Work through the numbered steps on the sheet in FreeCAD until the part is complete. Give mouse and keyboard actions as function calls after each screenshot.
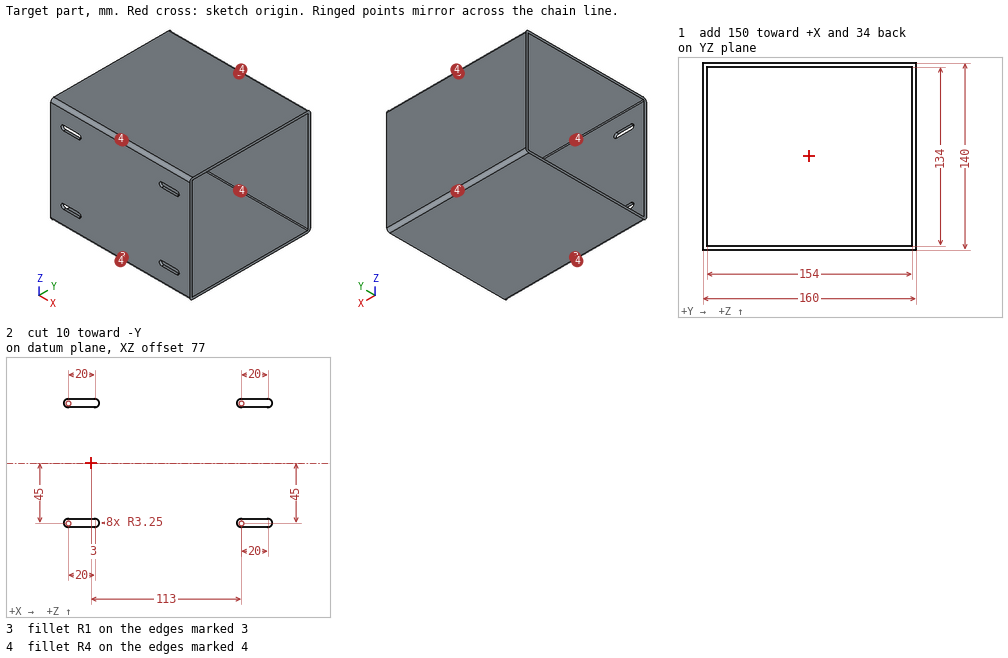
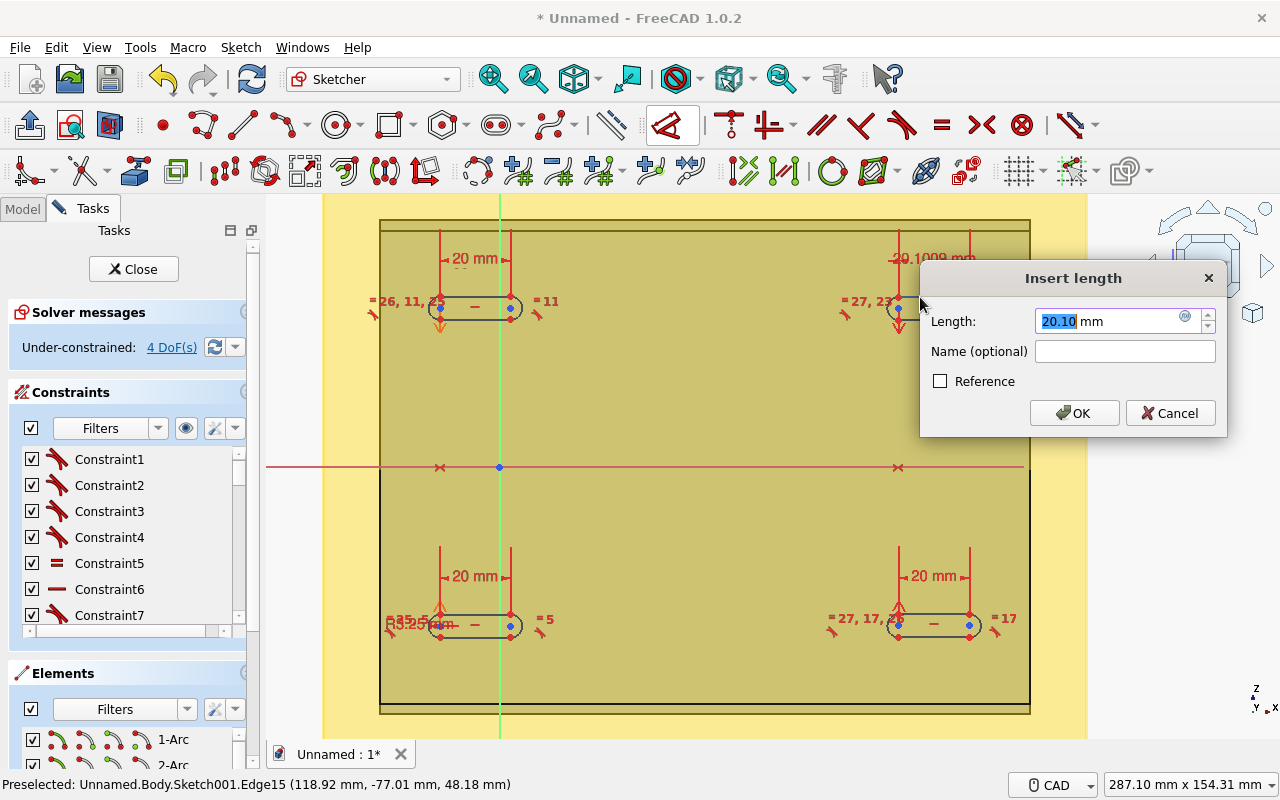
text(20)
key(Return)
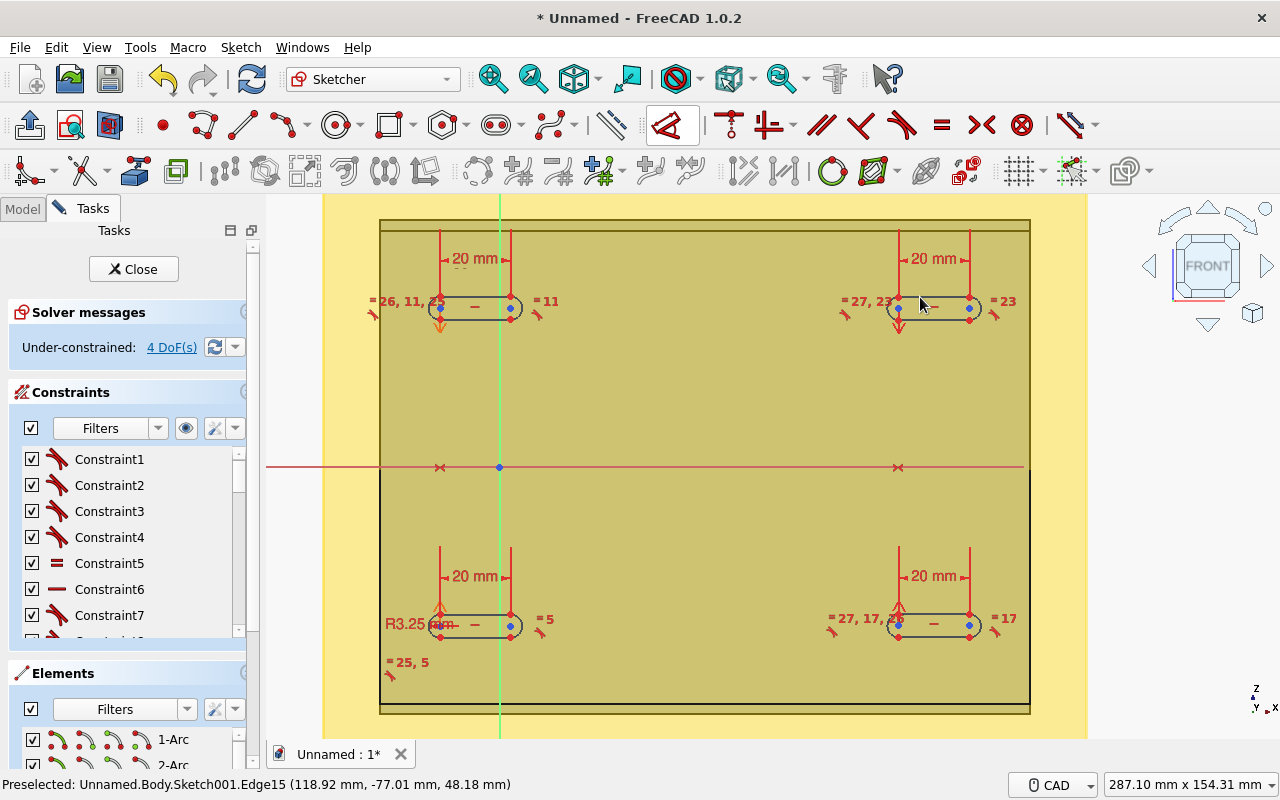
scroll(511, 638, up, 7)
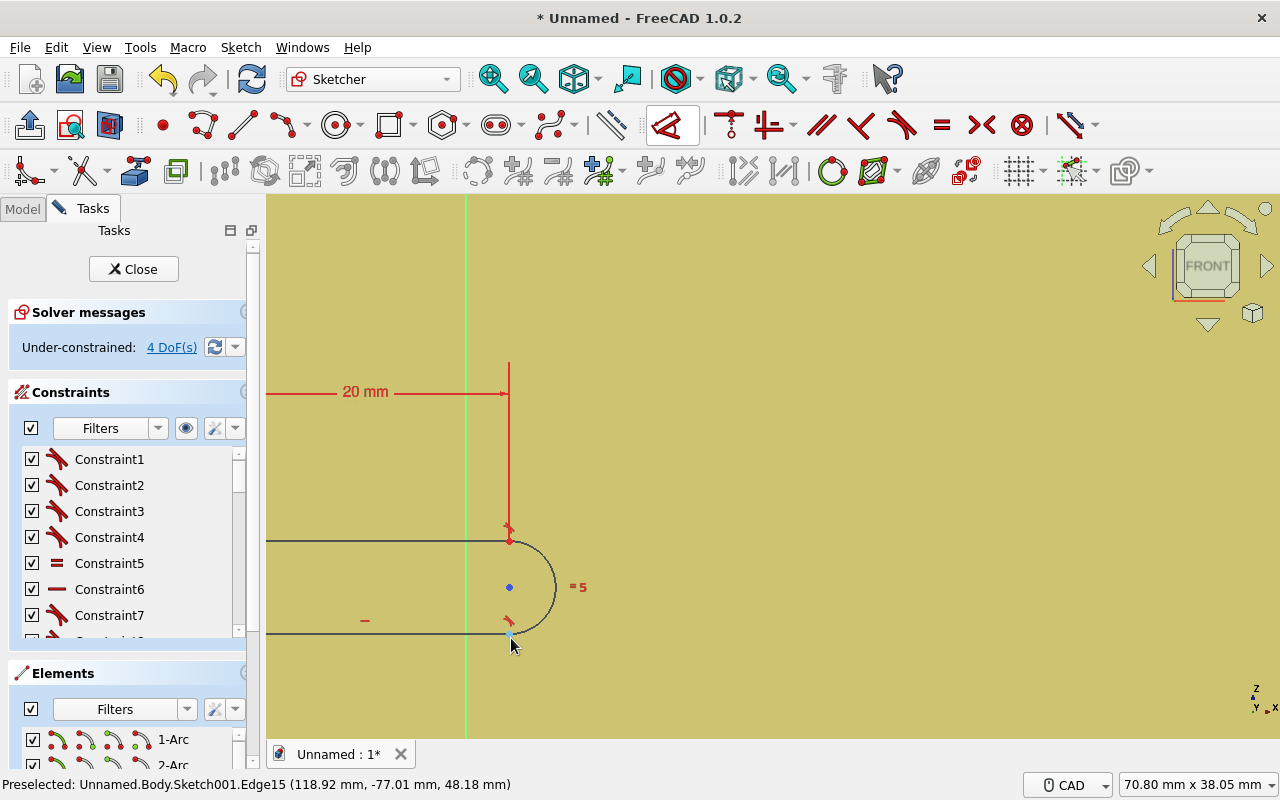
click(509, 634)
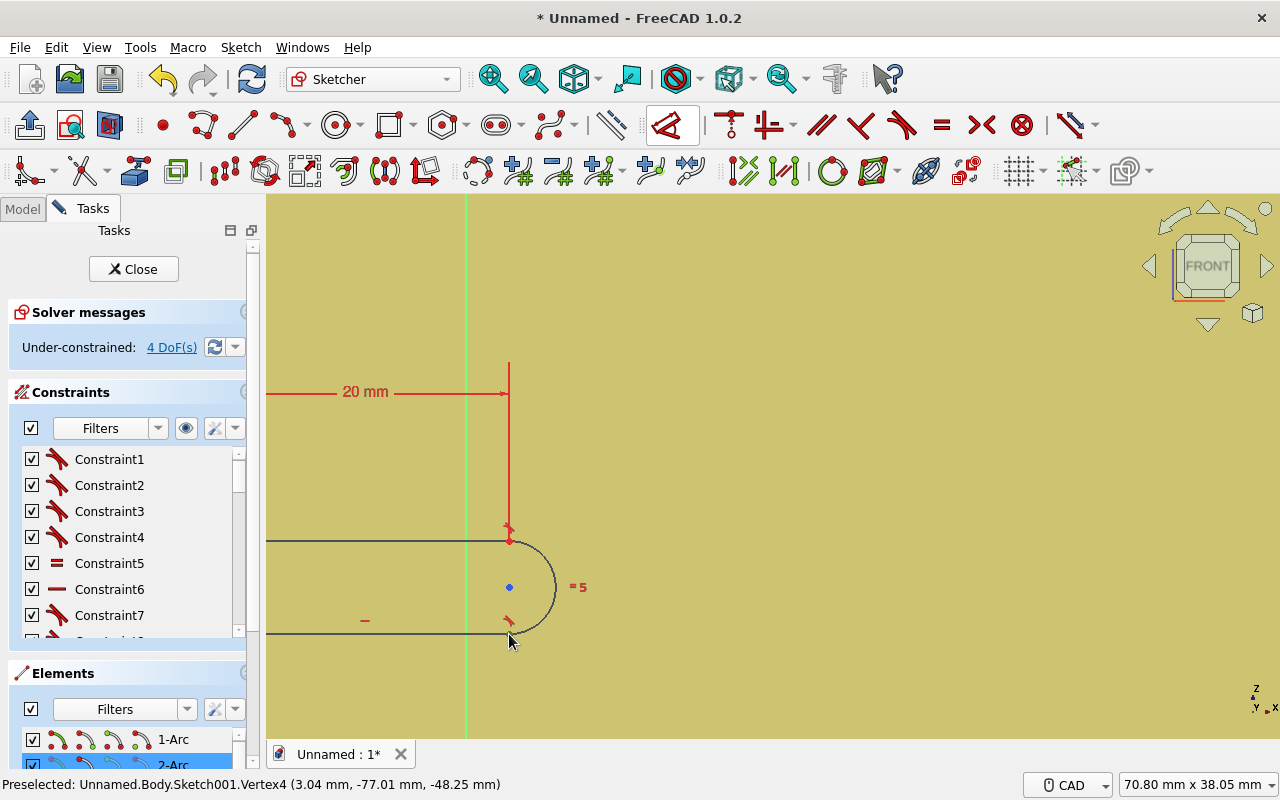
key(l)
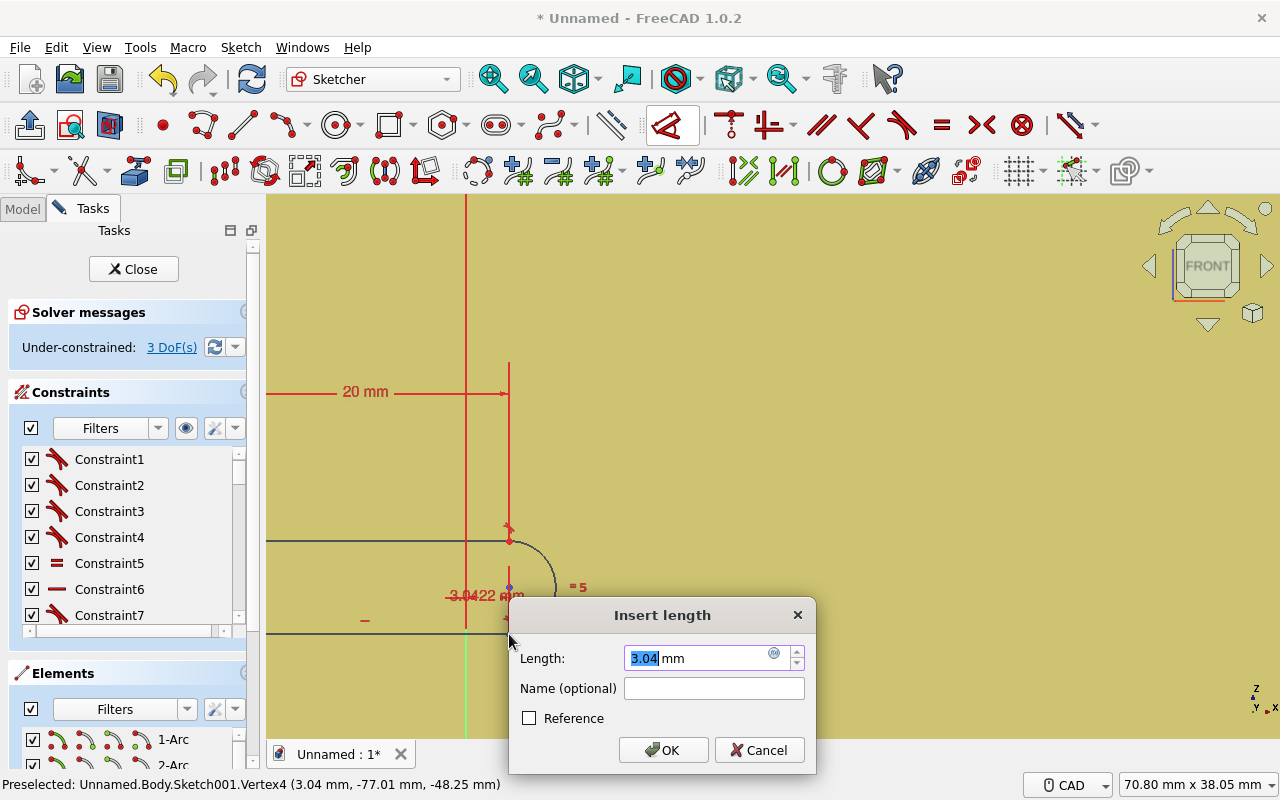
text(3)
key(Return)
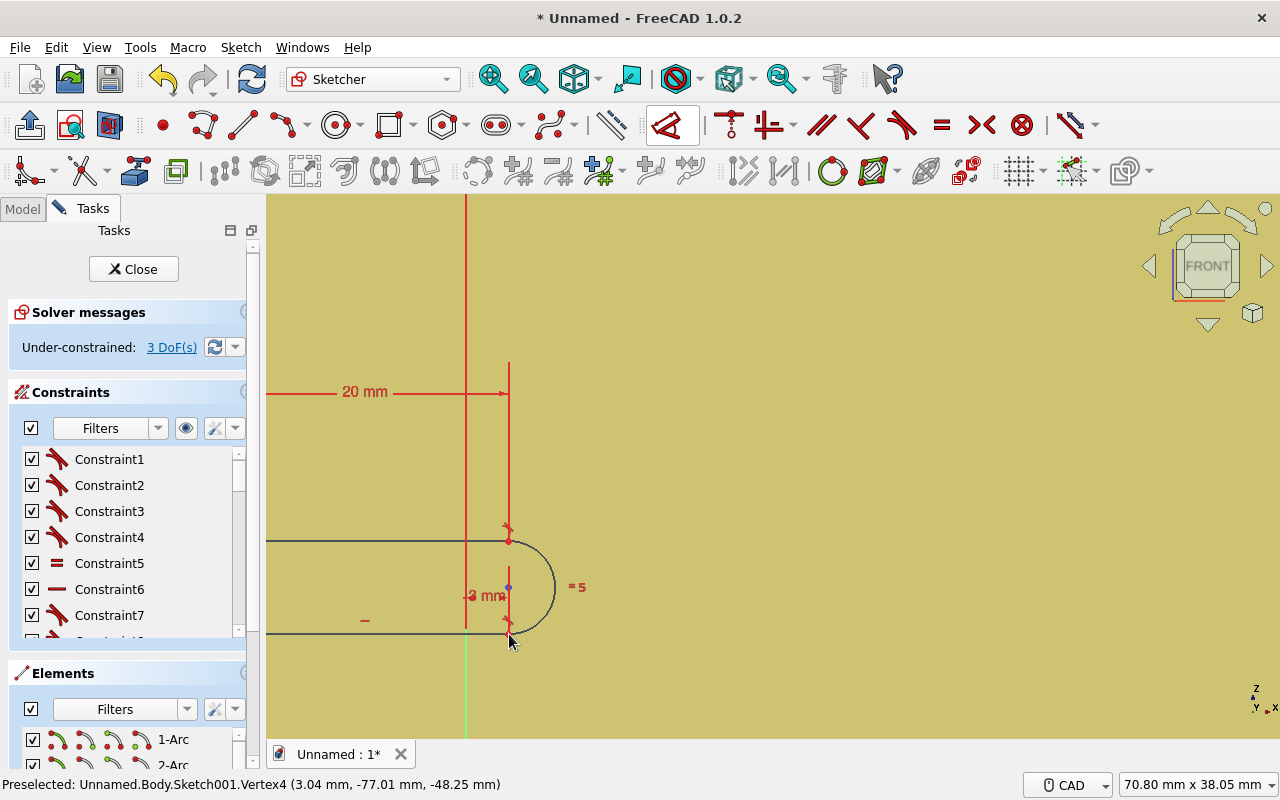
scroll(511, 638, down, 7)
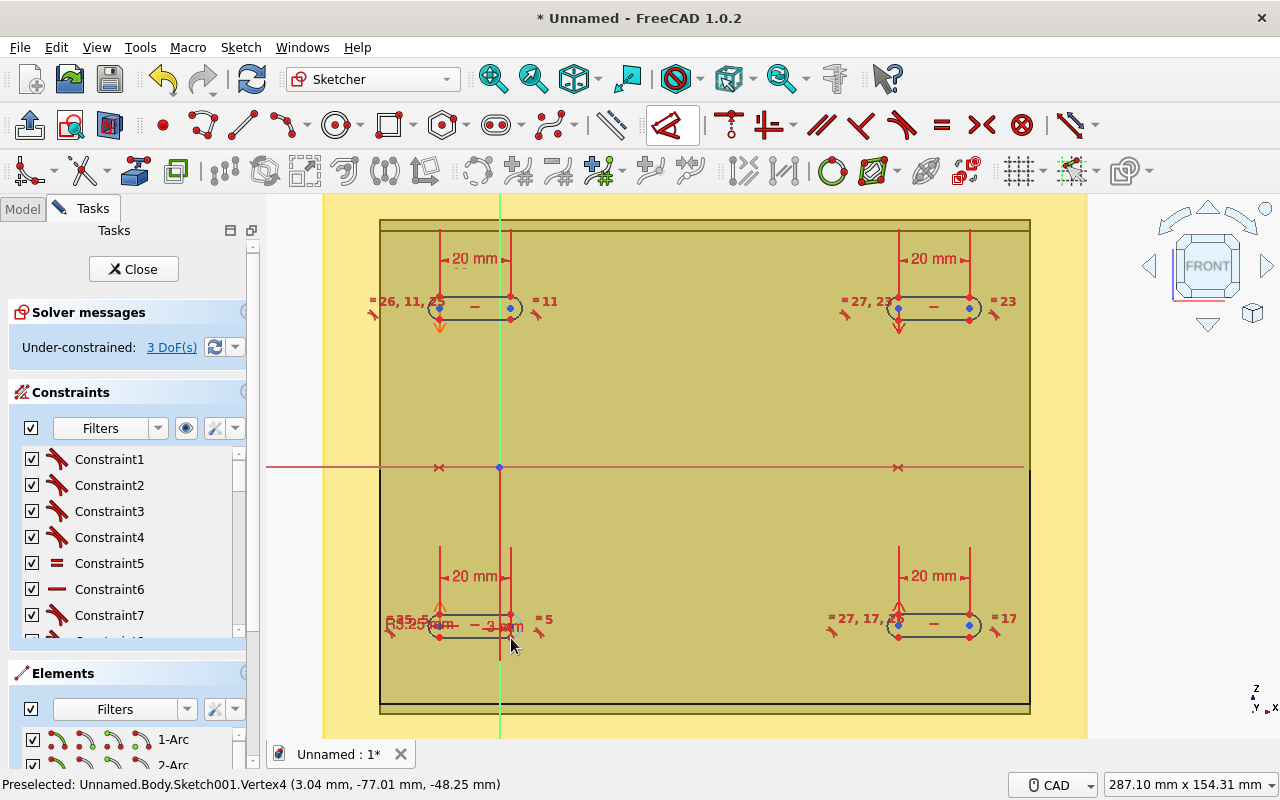
click(440, 626)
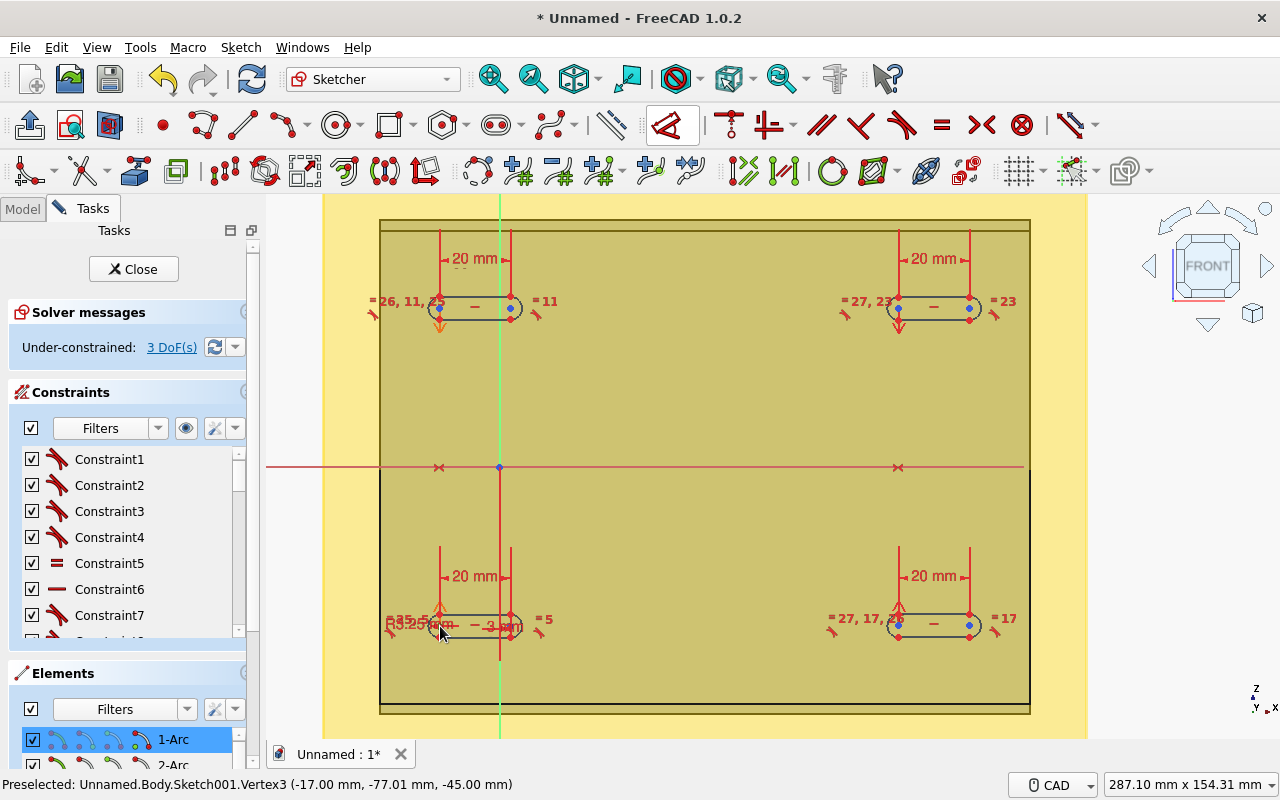
key(i)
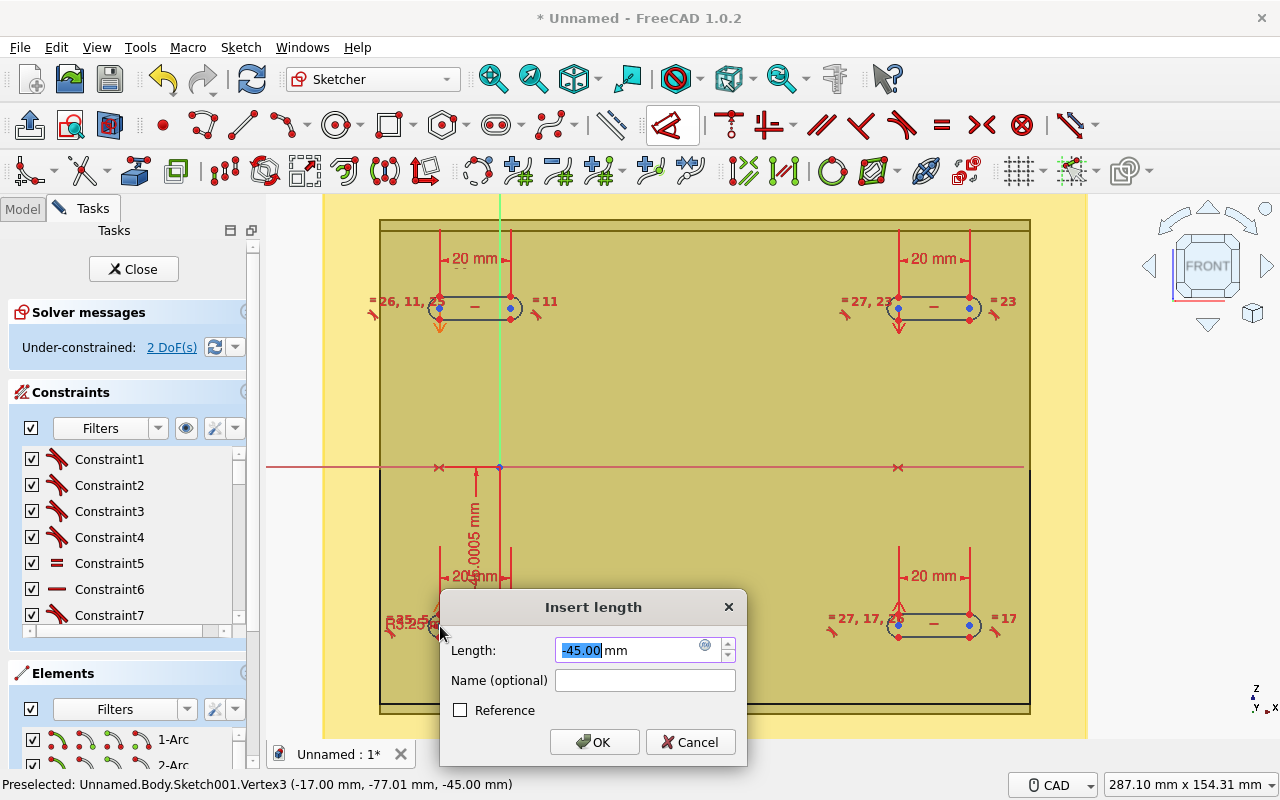
text(-45)
key(Return)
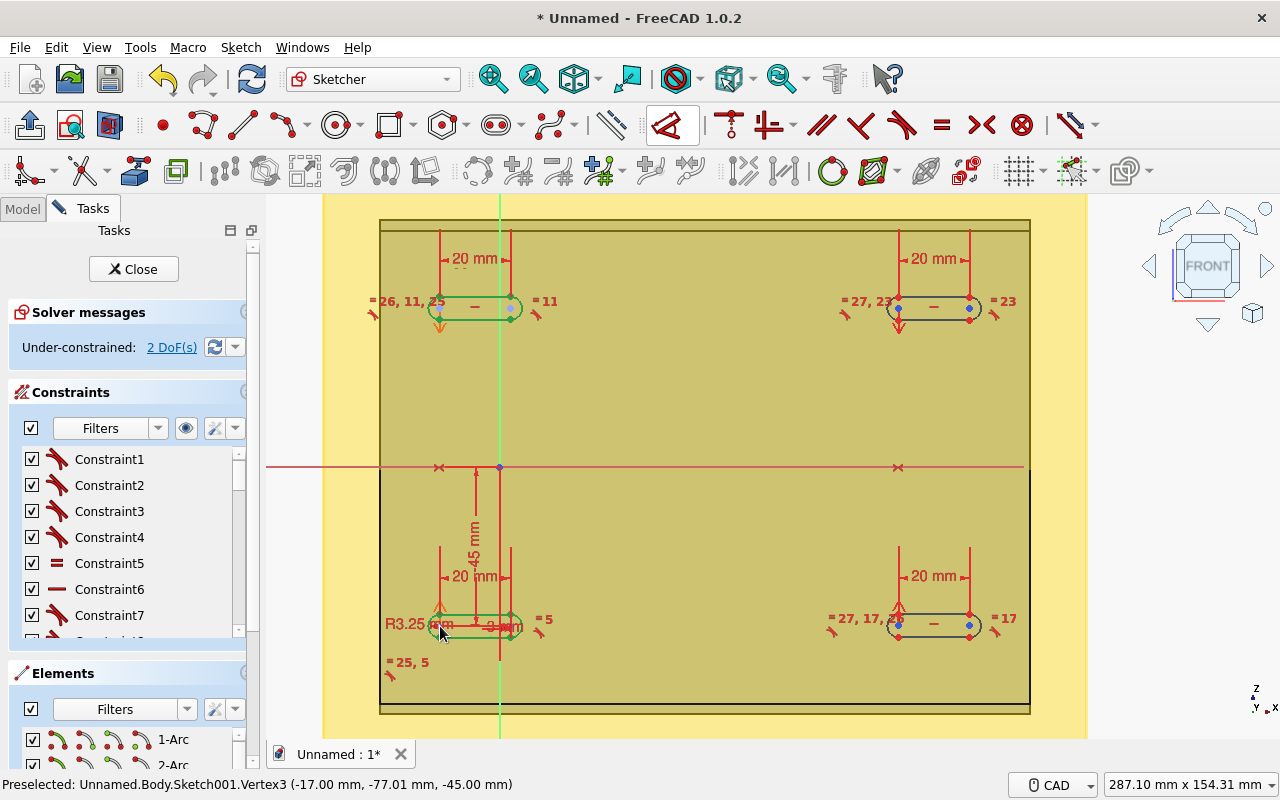
click(899, 626)